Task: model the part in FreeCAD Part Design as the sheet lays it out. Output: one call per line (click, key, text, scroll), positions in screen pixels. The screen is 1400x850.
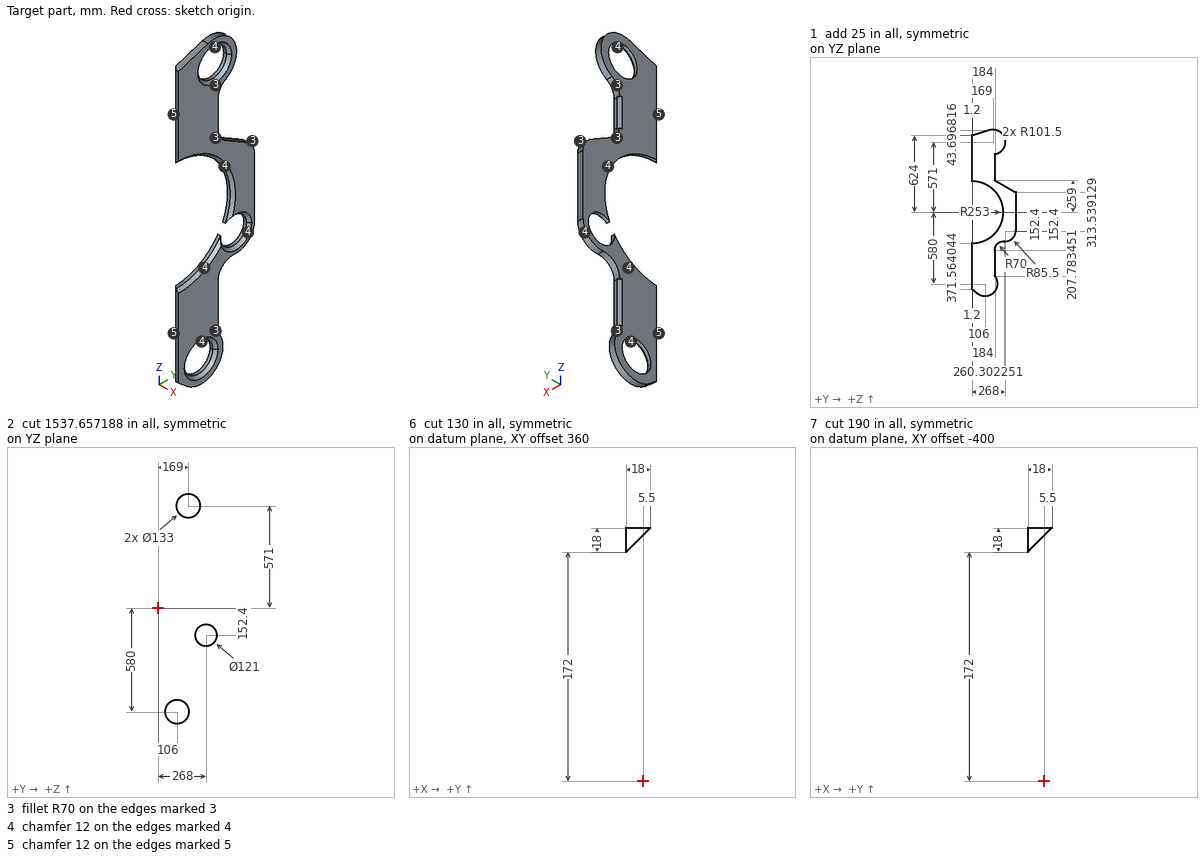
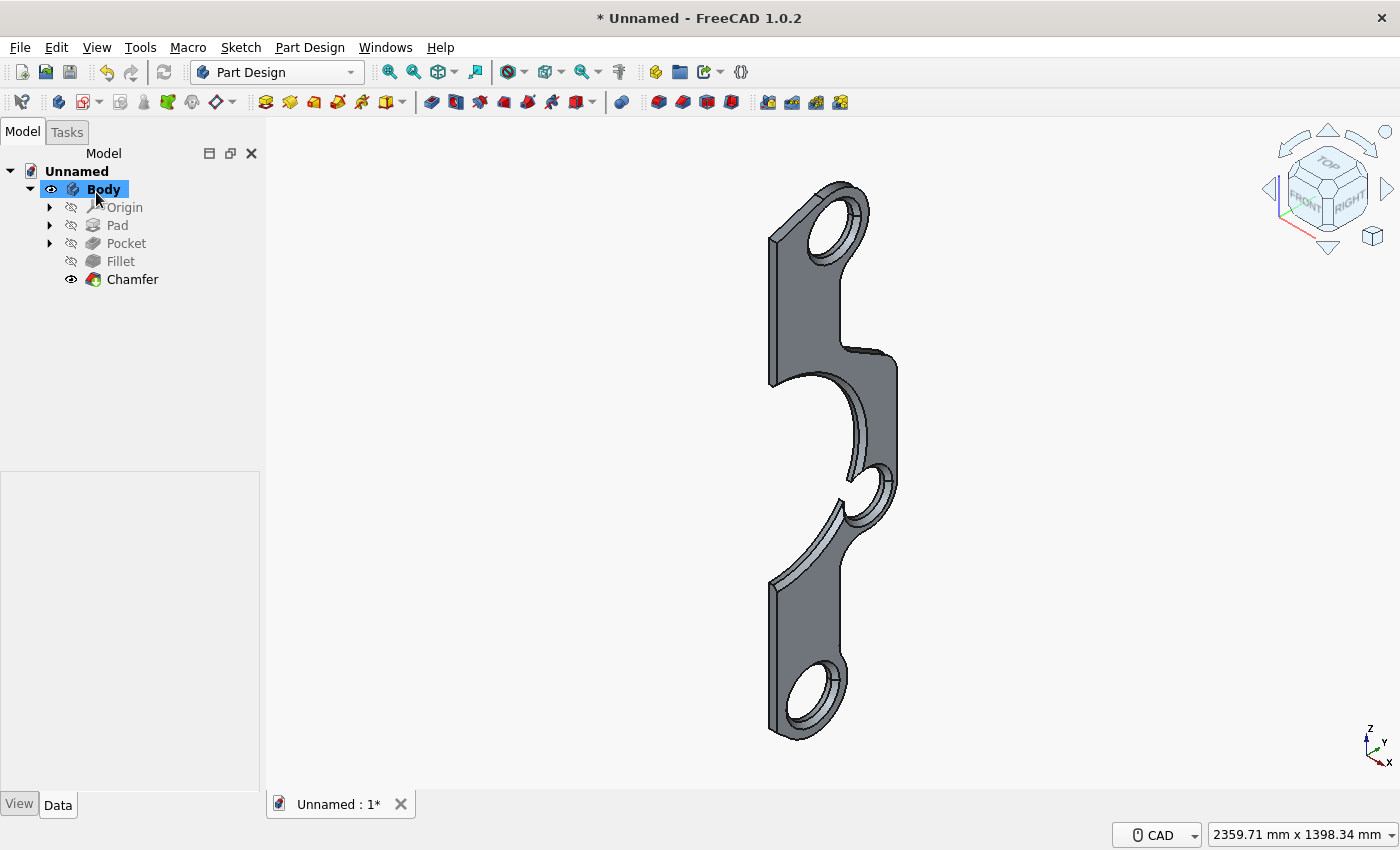
key(2)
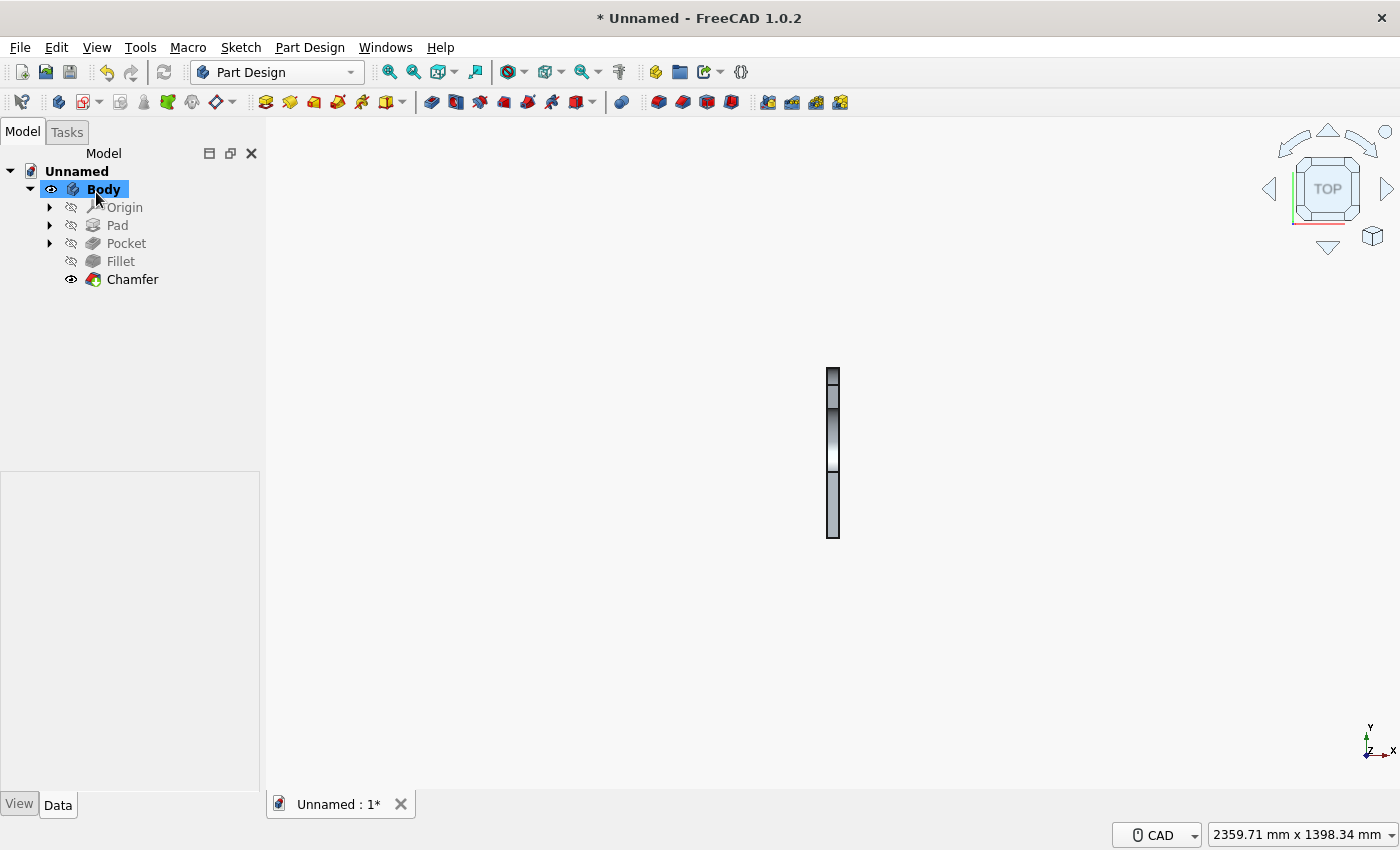
key(v)
key(f)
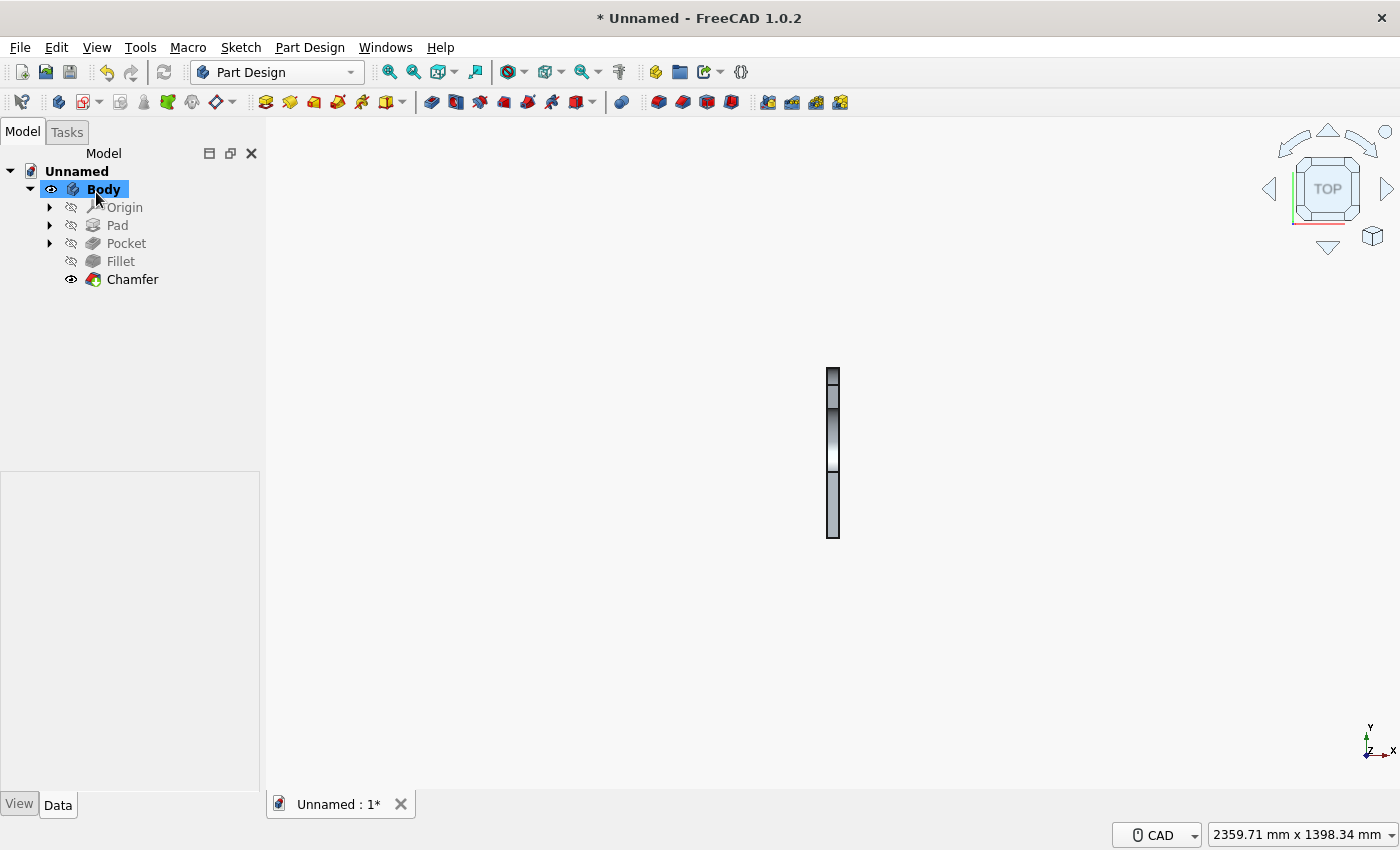
key(0)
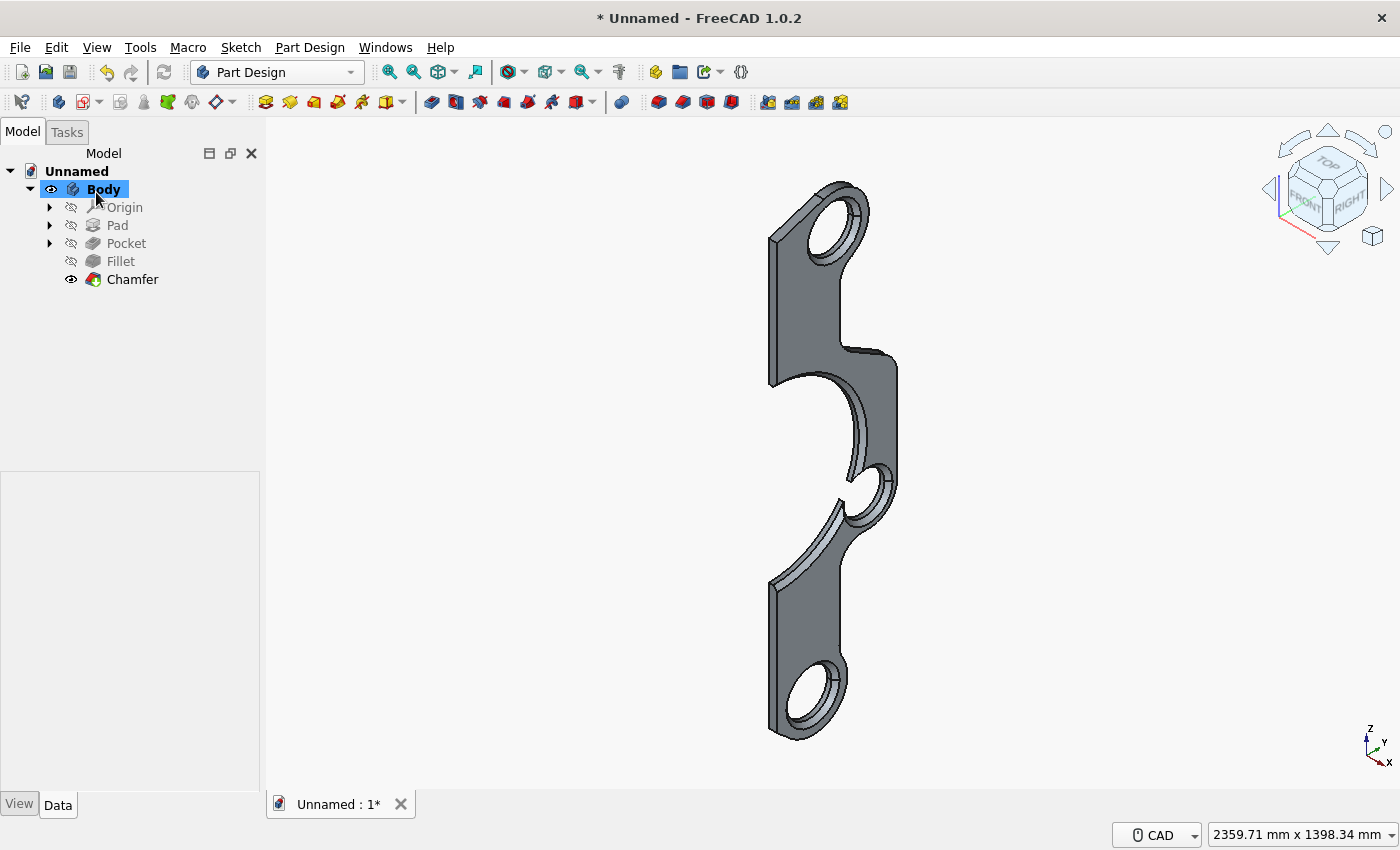
key(1)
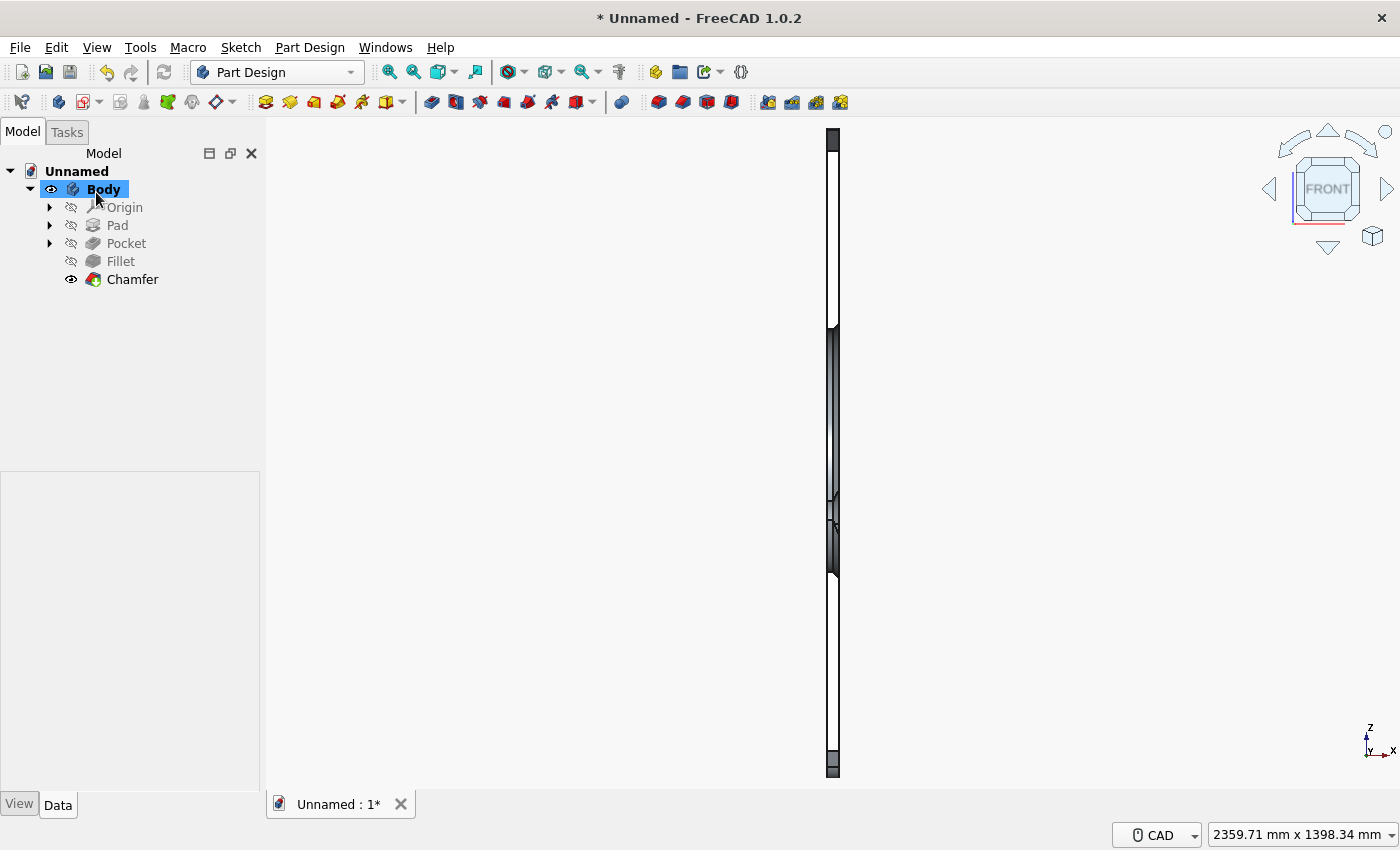
click(827, 661)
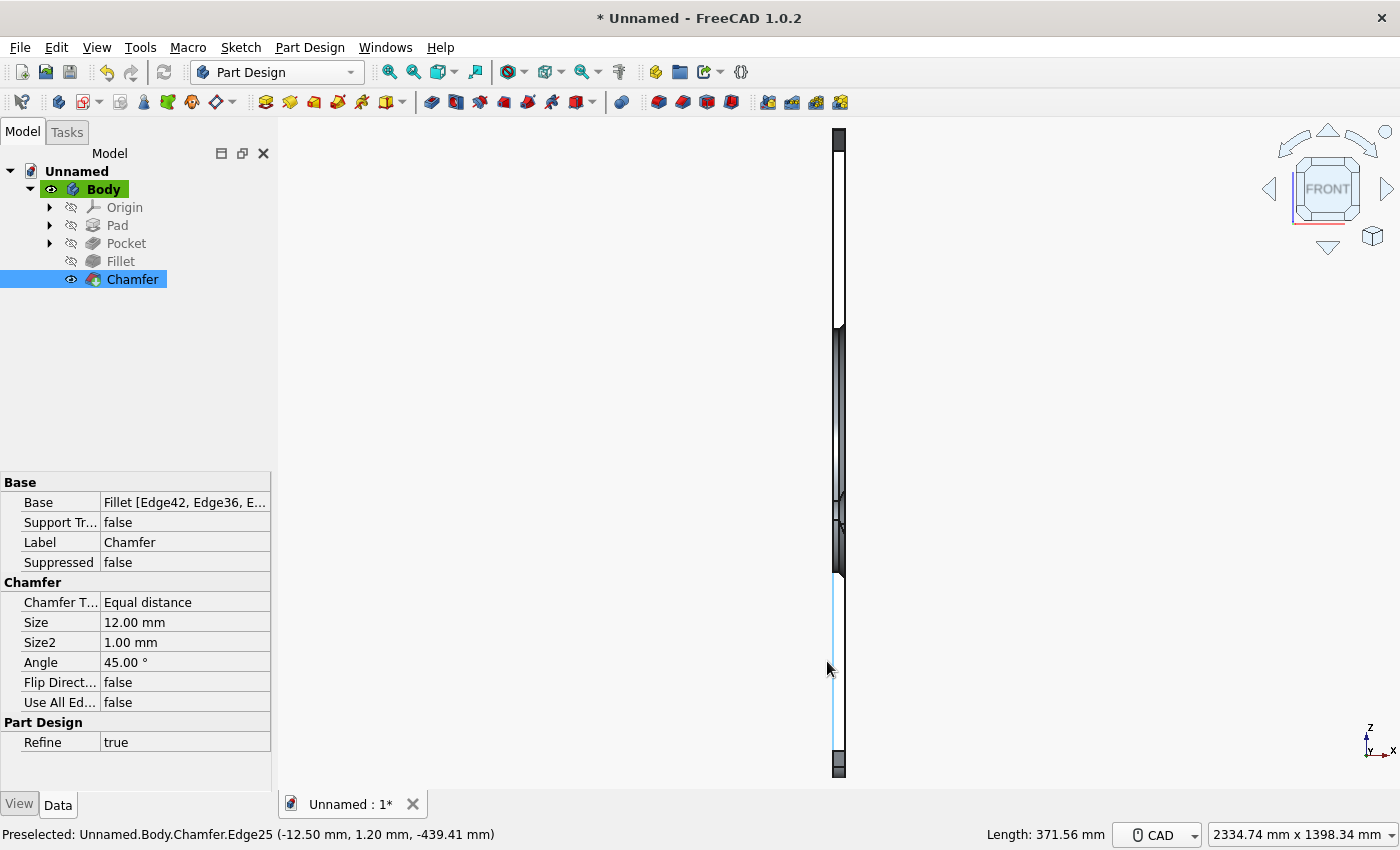
click(833, 239, ctrl)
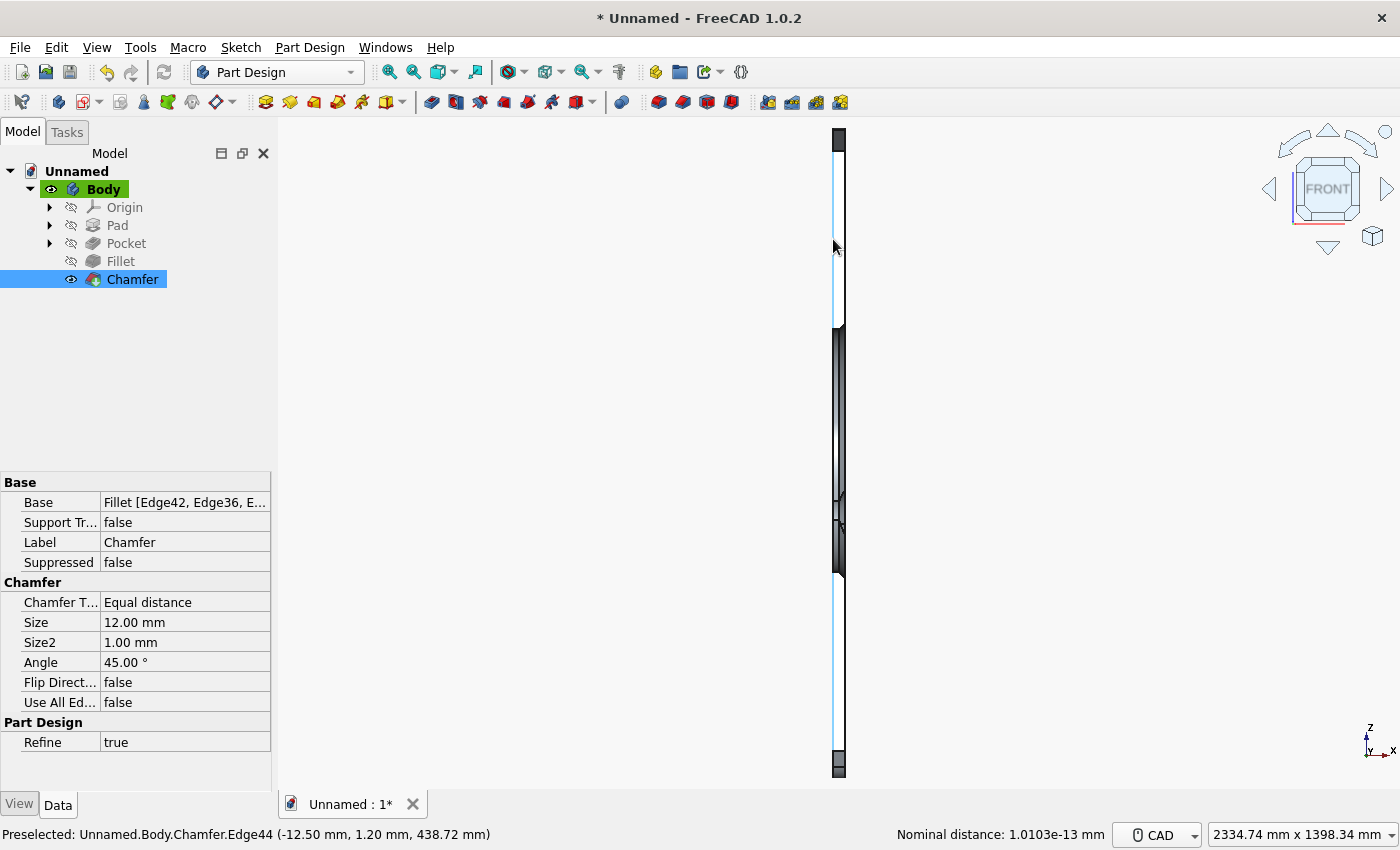
click(684, 102)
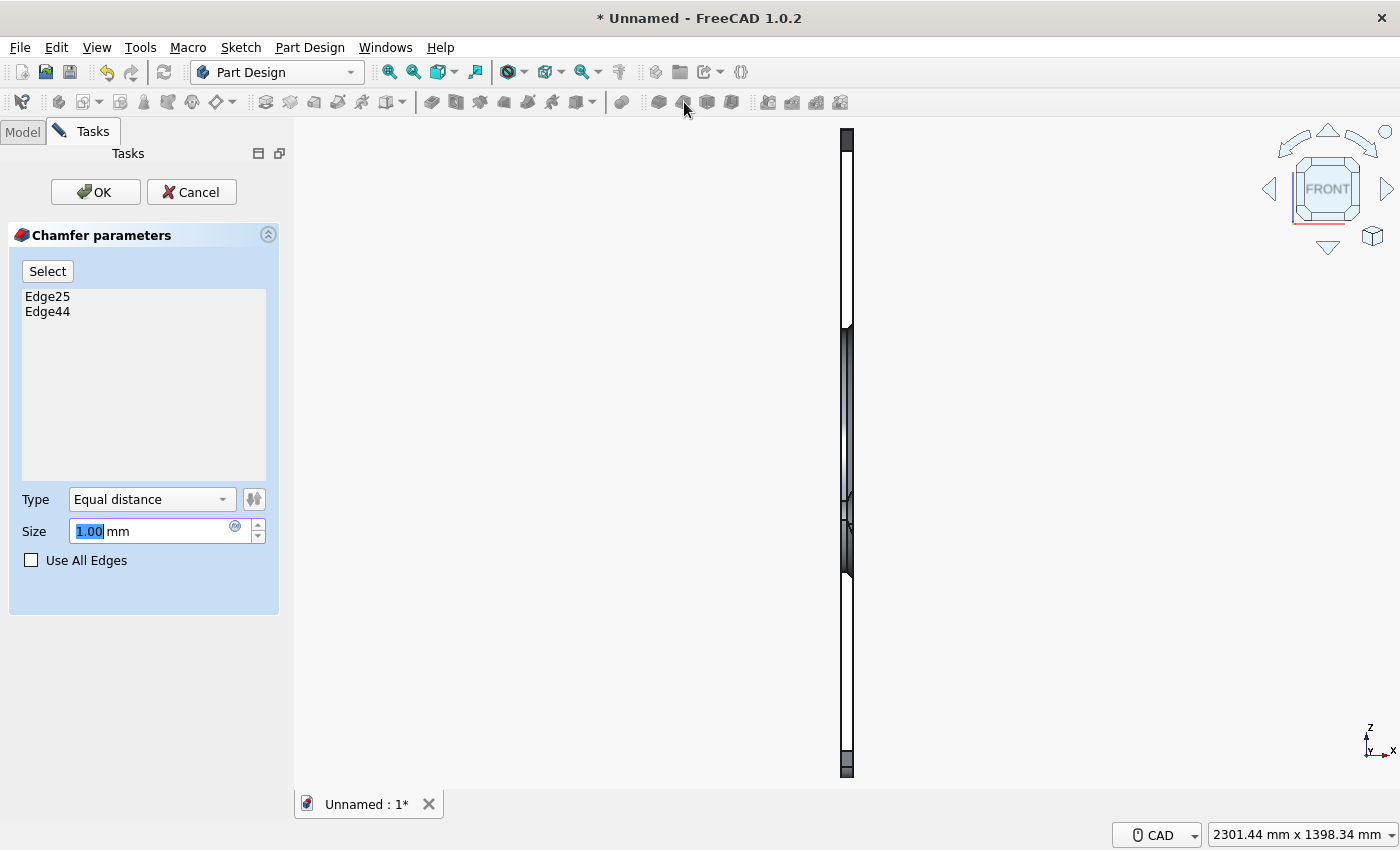
text(12)
key(Tab)